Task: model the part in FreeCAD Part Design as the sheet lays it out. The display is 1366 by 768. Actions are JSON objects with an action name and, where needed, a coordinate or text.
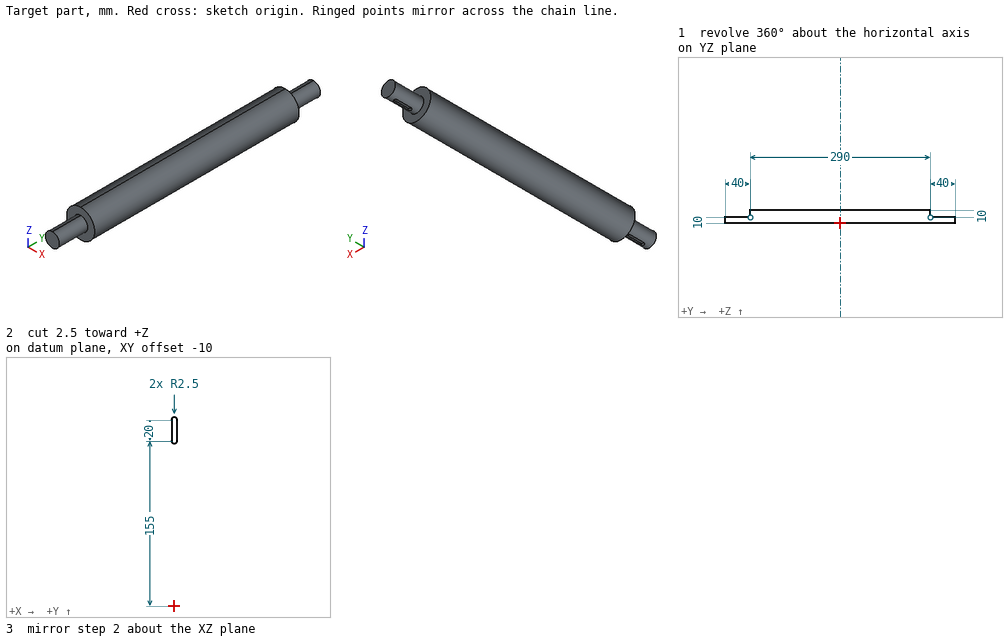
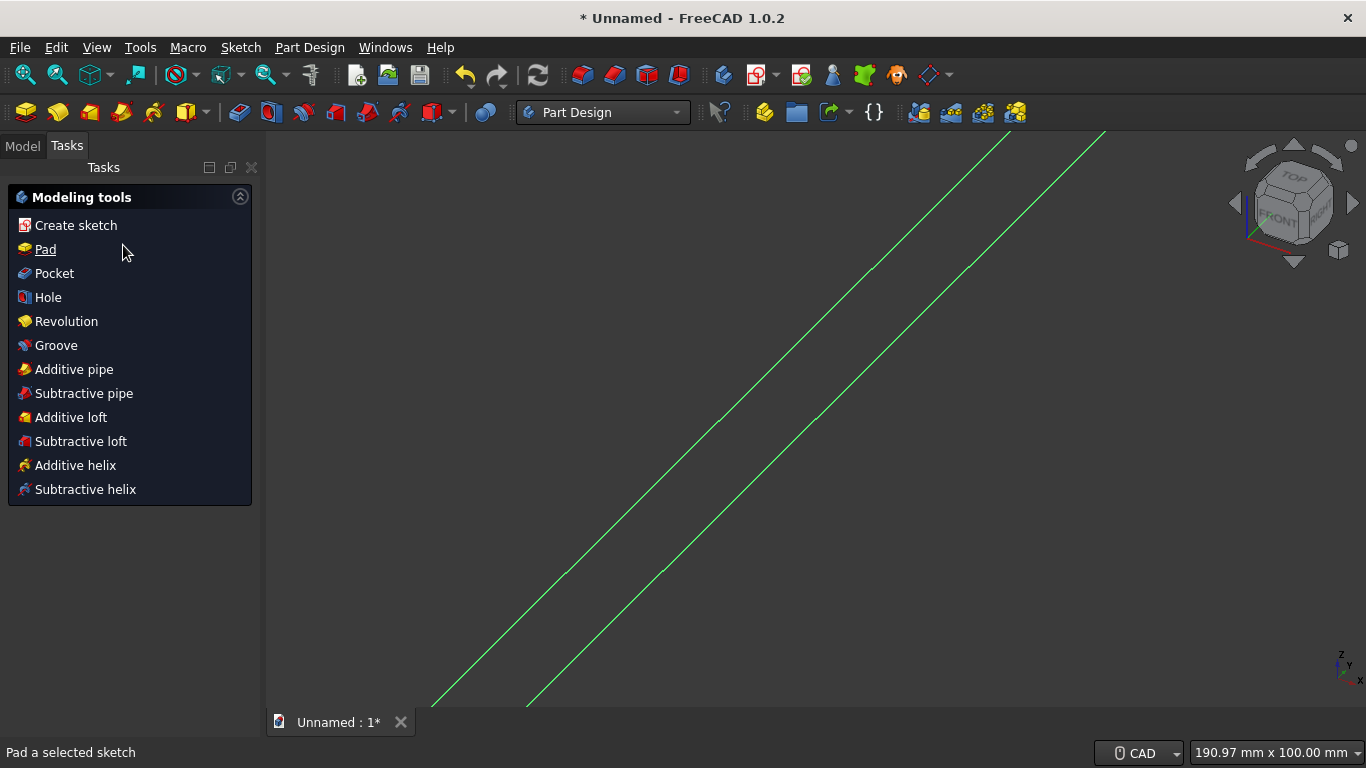
{"action": "left_click", "coordinate": [58, 112]}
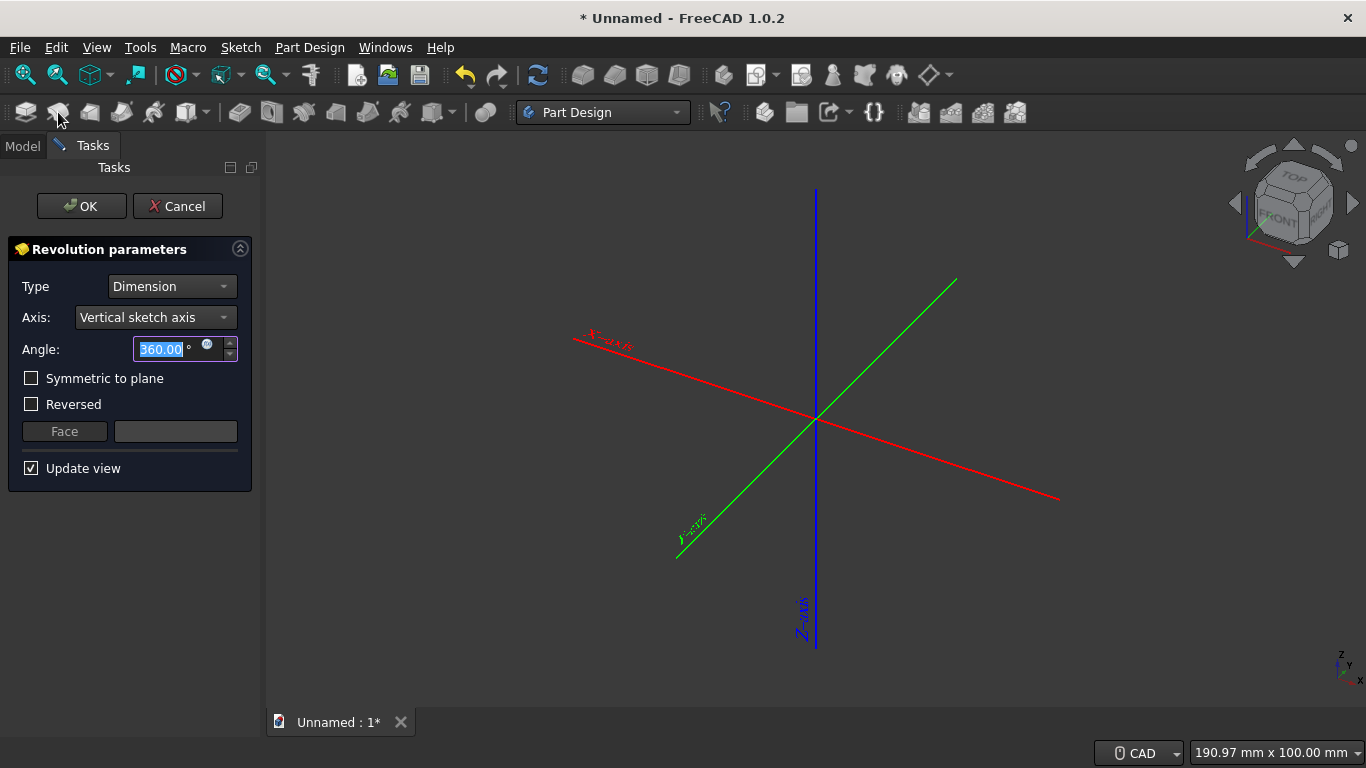
{"action": "left_click", "coordinate": [156, 318]}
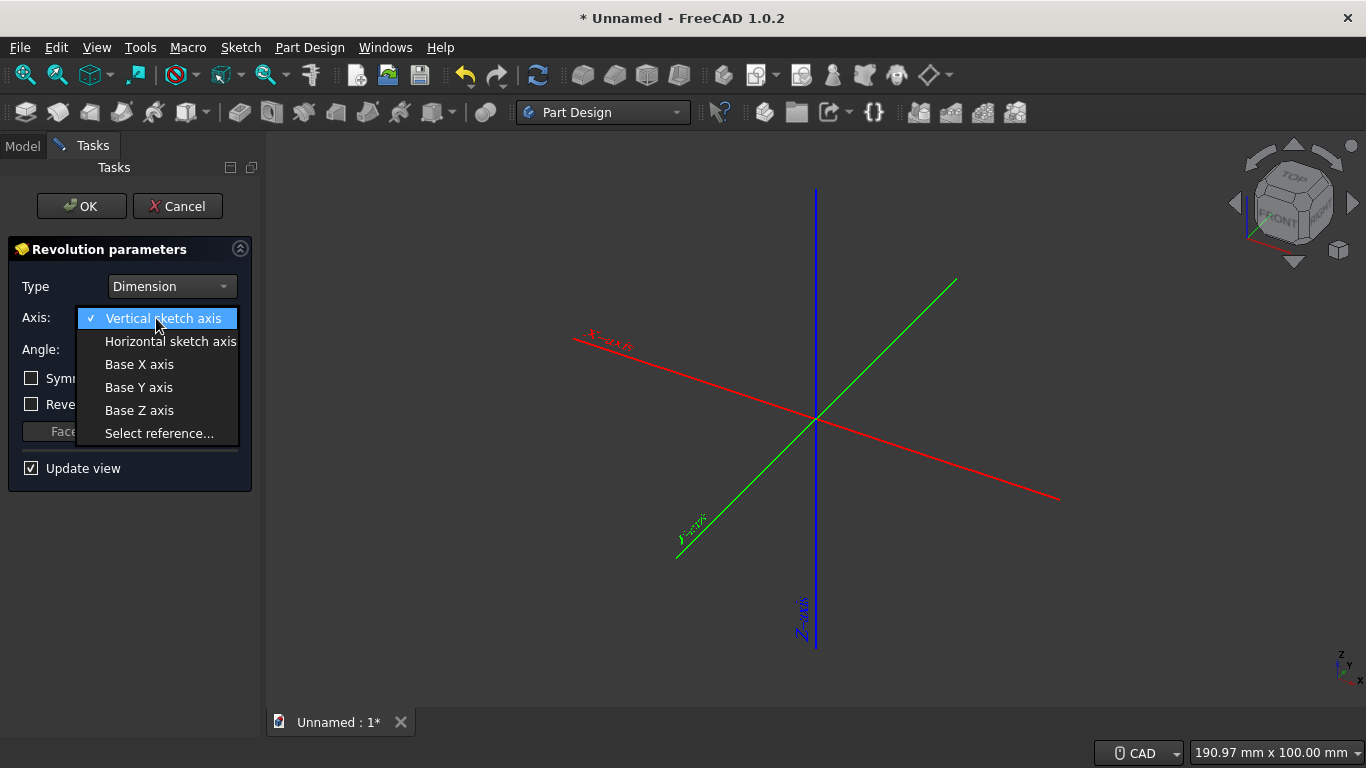
{"action": "left_click", "coordinate": [156, 342]}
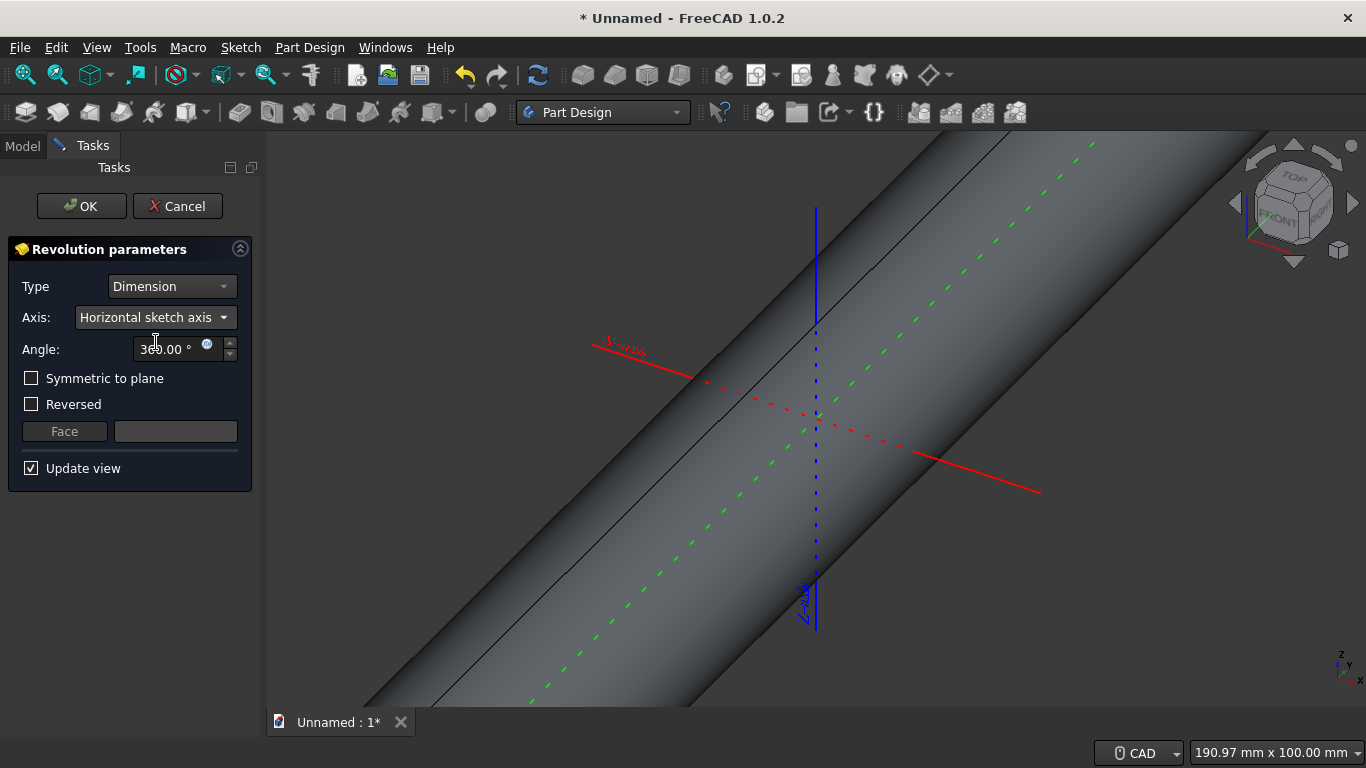
{"action": "left_click", "coordinate": [82, 206]}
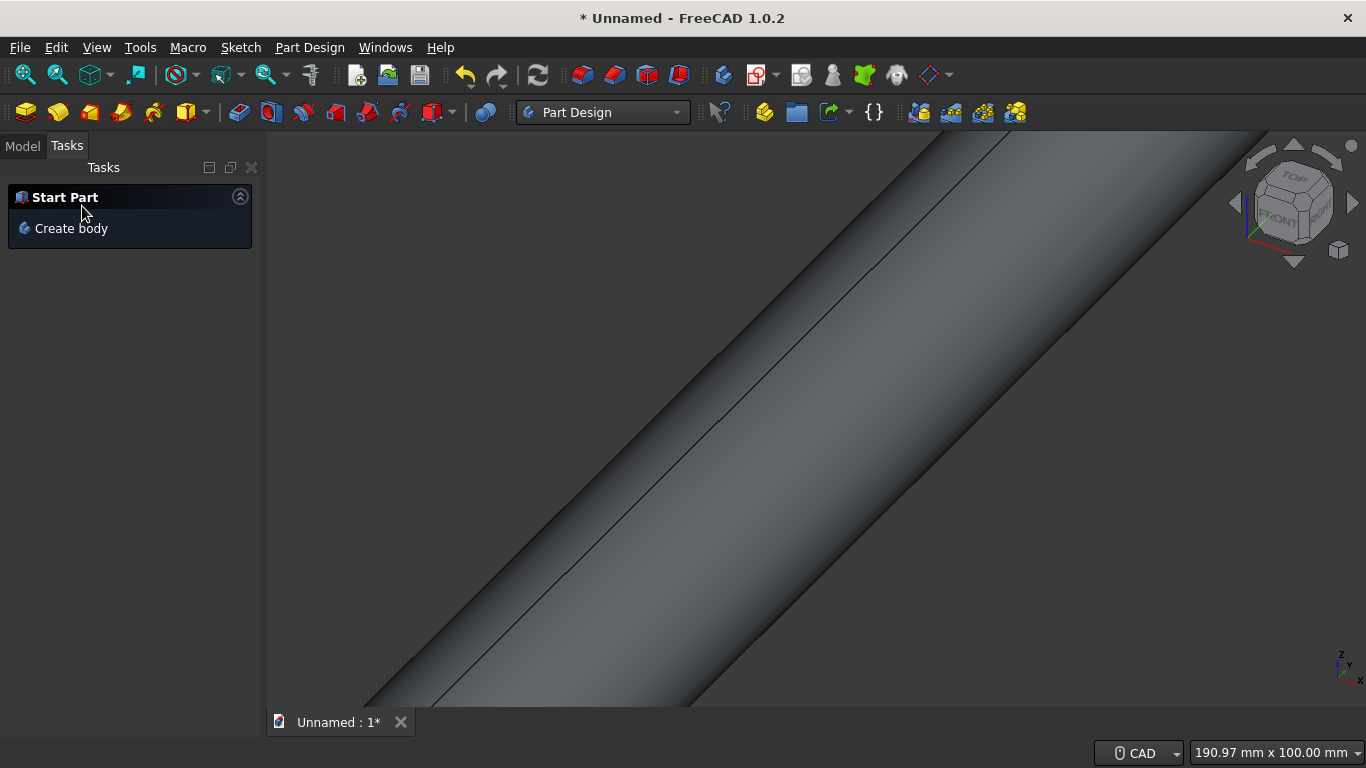
{"action": "left_click", "coordinate": [26, 76]}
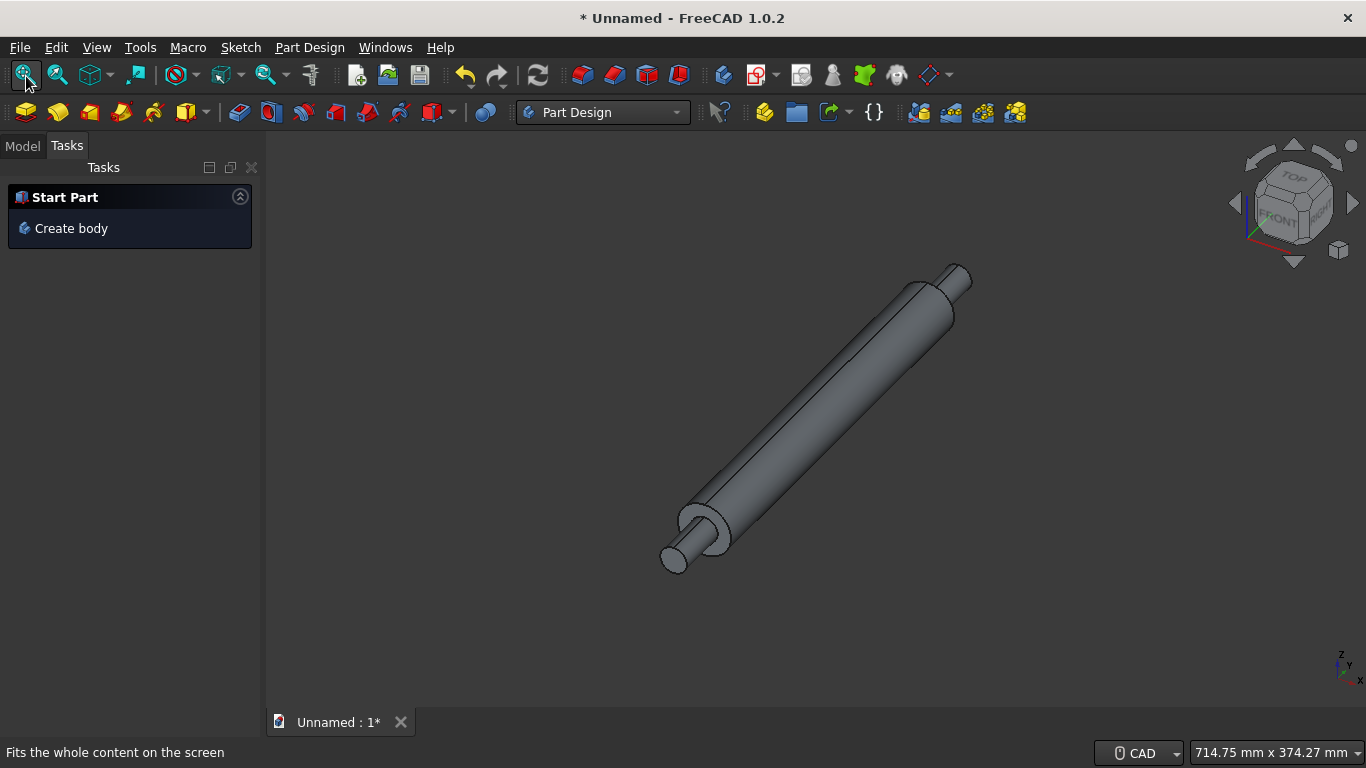
{"action": "left_click", "coordinate": [23, 145]}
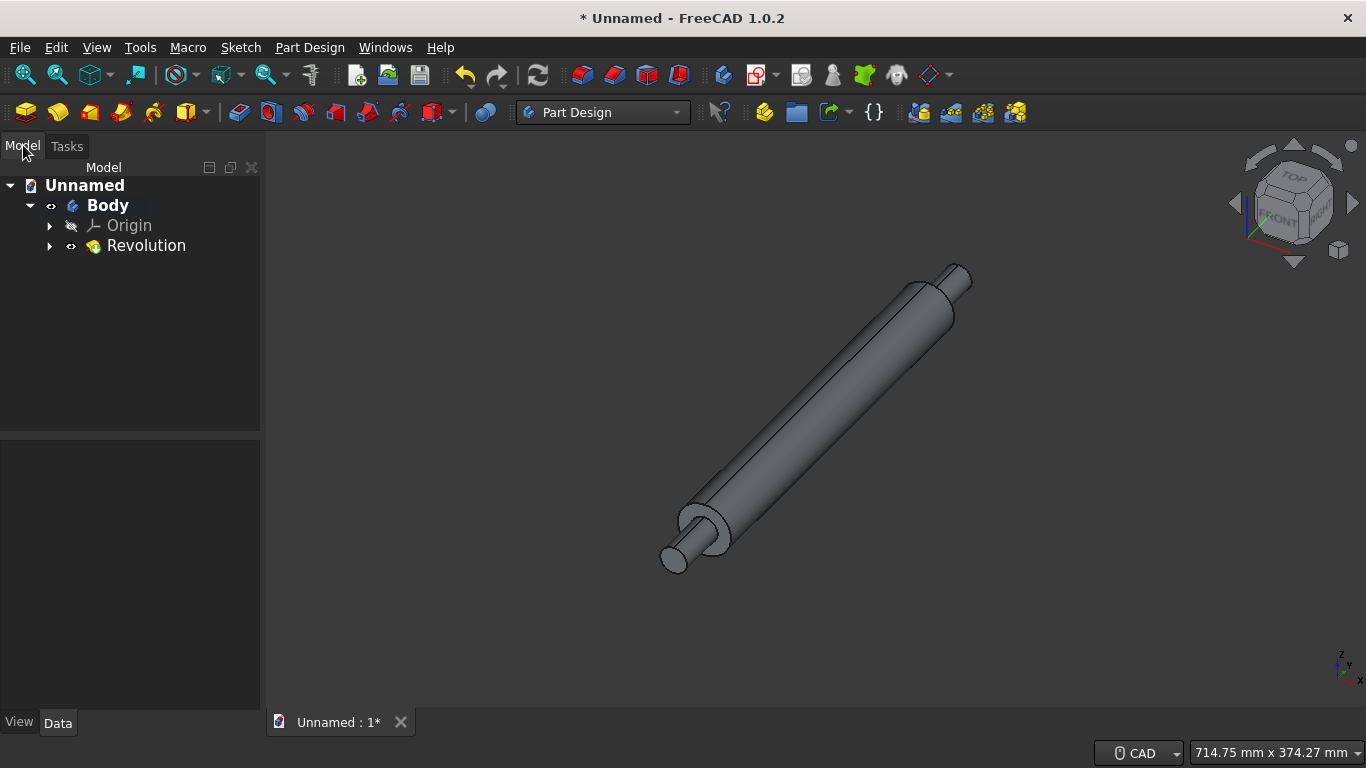
{"action": "left_click", "coordinate": [50, 226]}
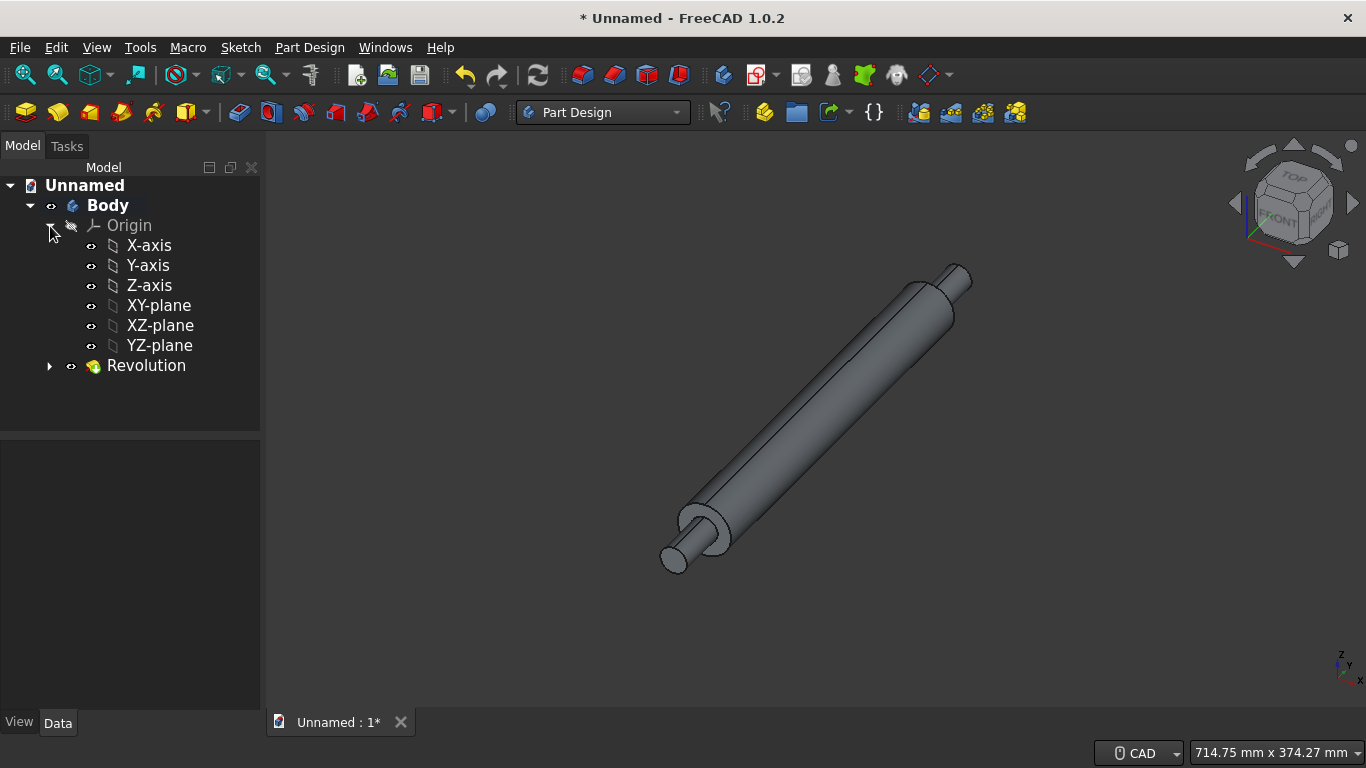
{"action": "left_click", "coordinate": [136, 306]}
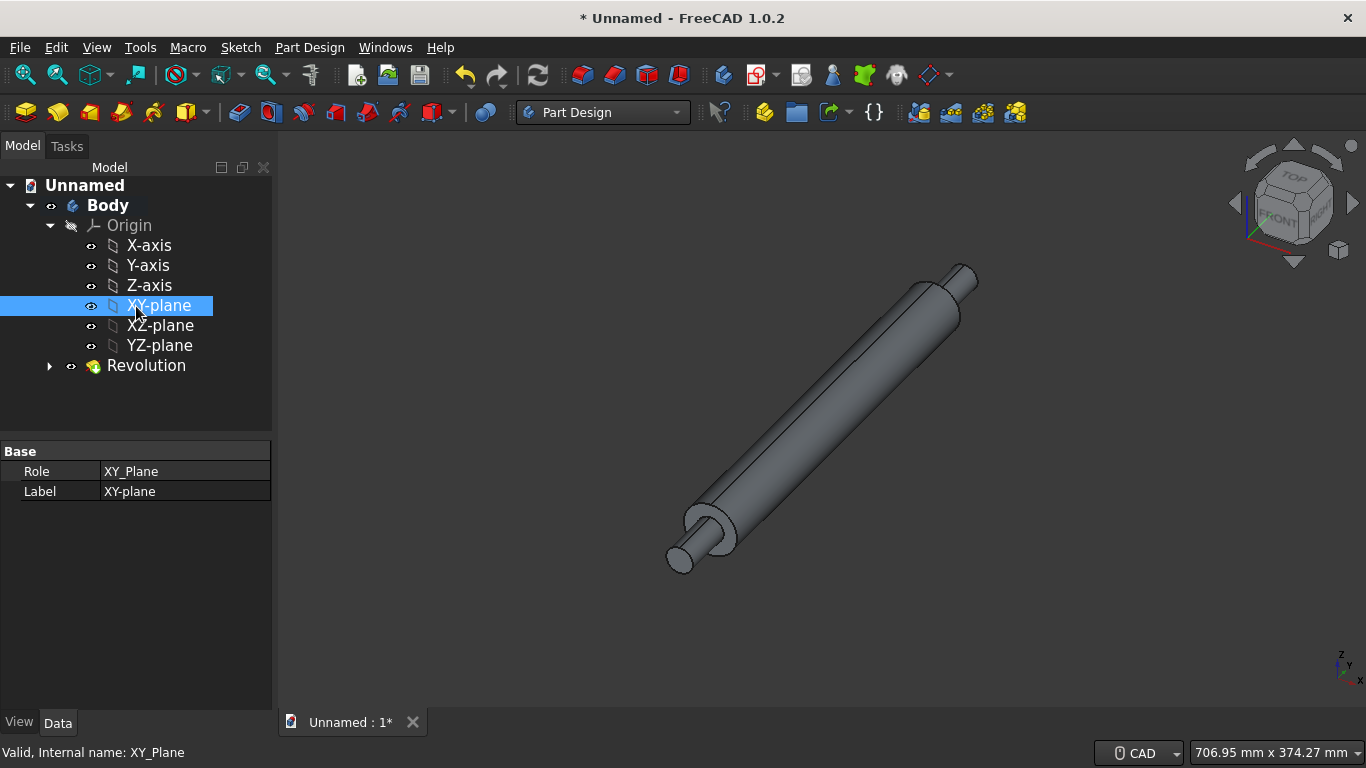
{"action": "left_click", "coordinate": [930, 76]}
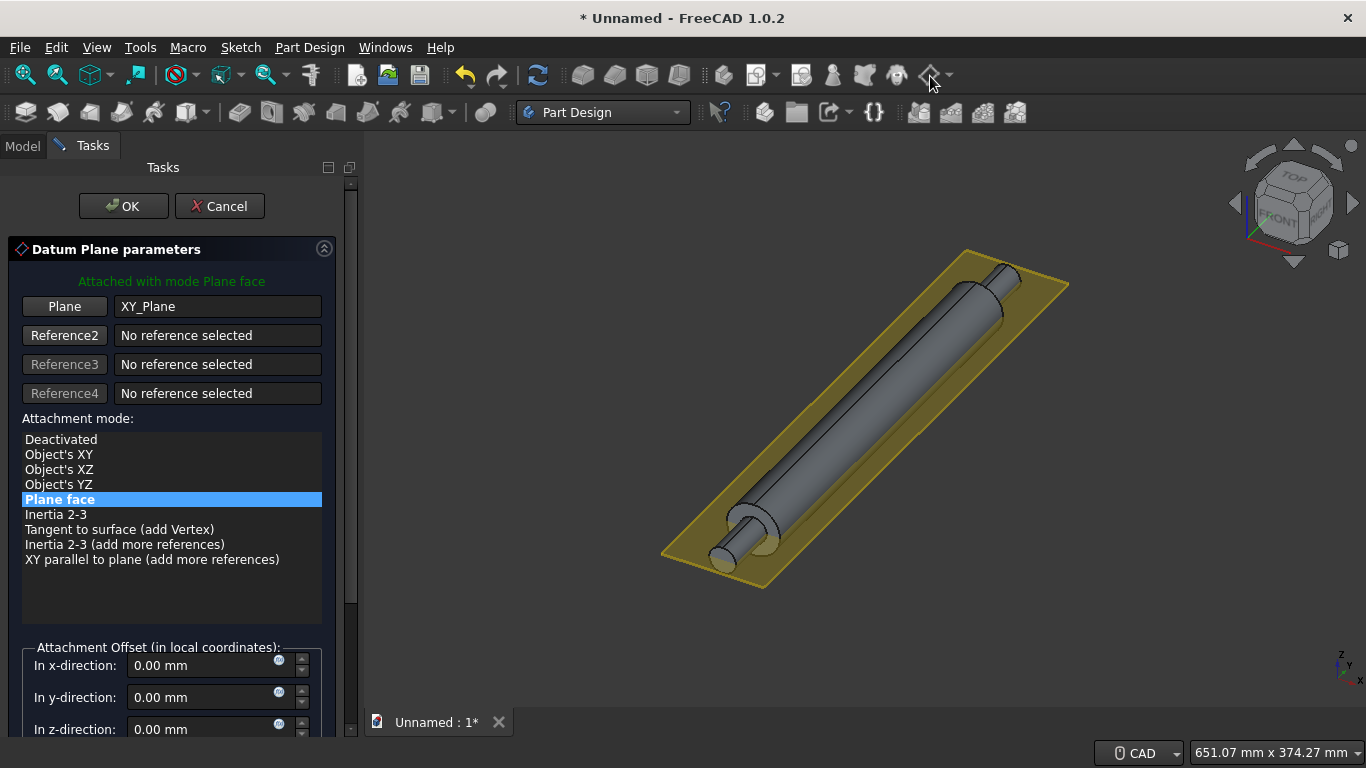
{"action": "scroll", "coordinate": [351, 456], "scroll_direction": "down", "scroll_amount": 2}